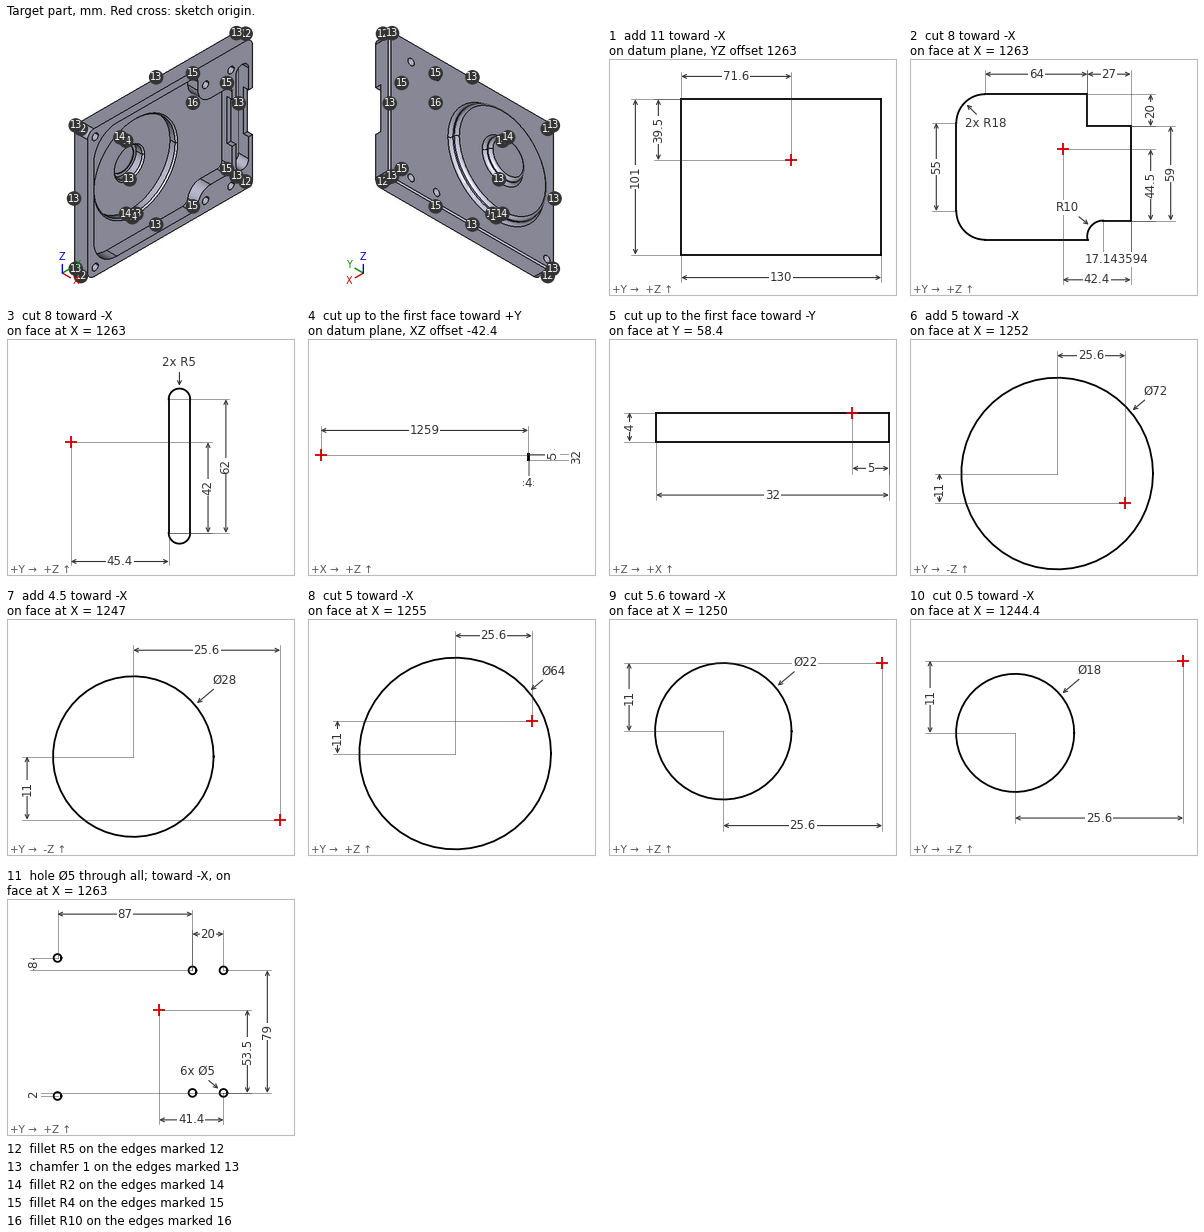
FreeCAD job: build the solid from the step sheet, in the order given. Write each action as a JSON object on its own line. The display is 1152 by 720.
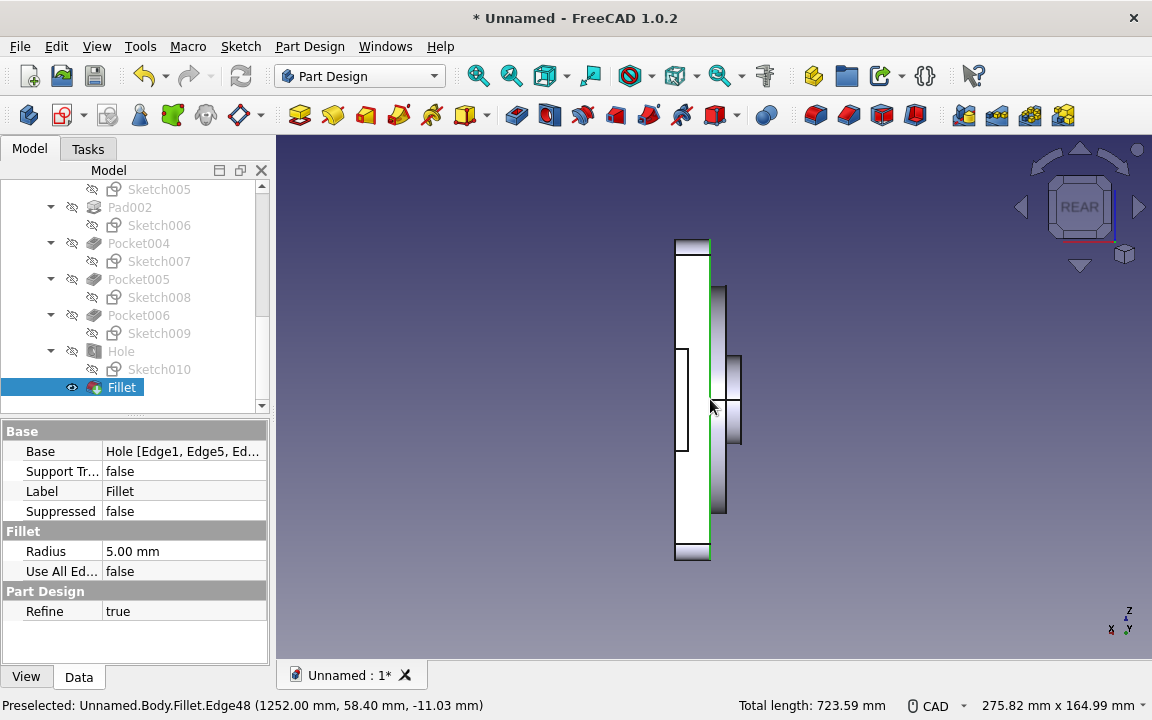
{"action": "left_click", "coordinate": [849, 116]}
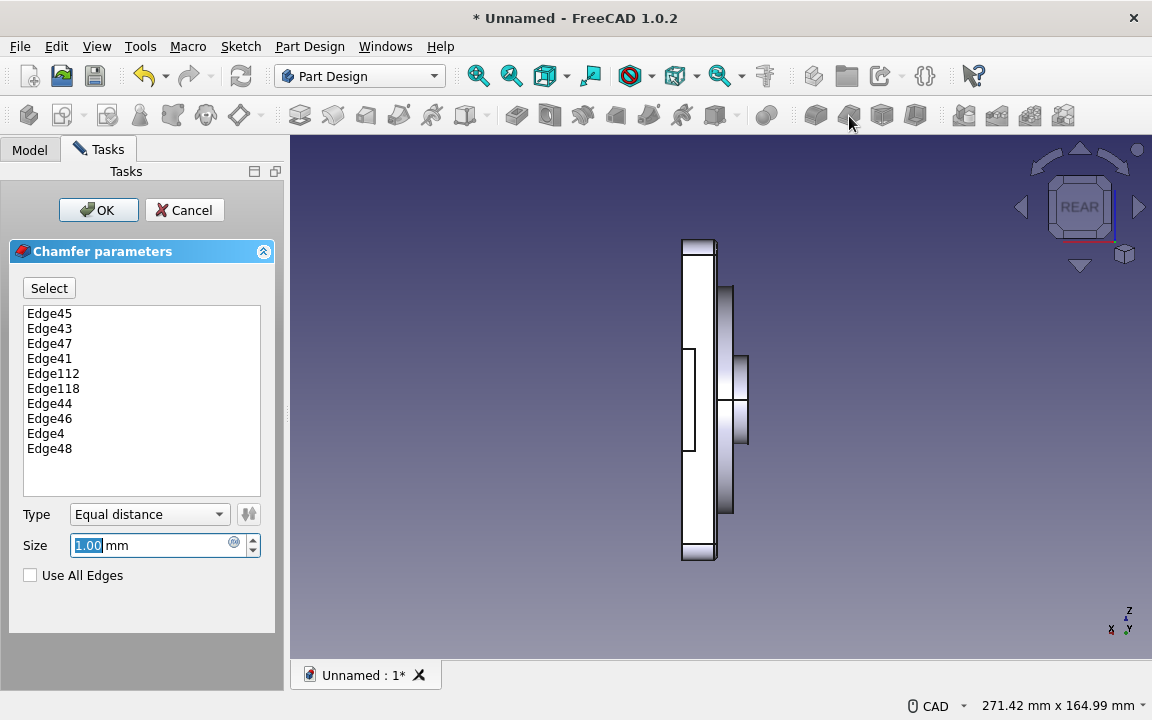
{"action": "type", "text": "1"}
{"action": "key", "text": "Tab"}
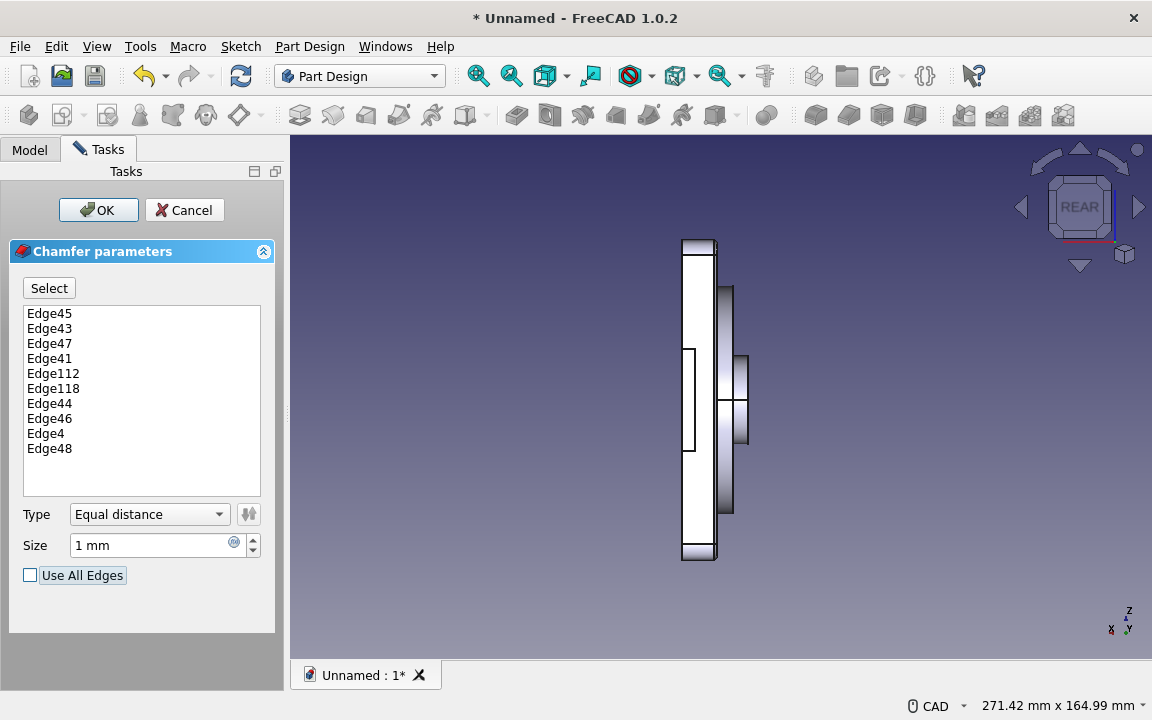
{"action": "left_click", "coordinate": [99, 210]}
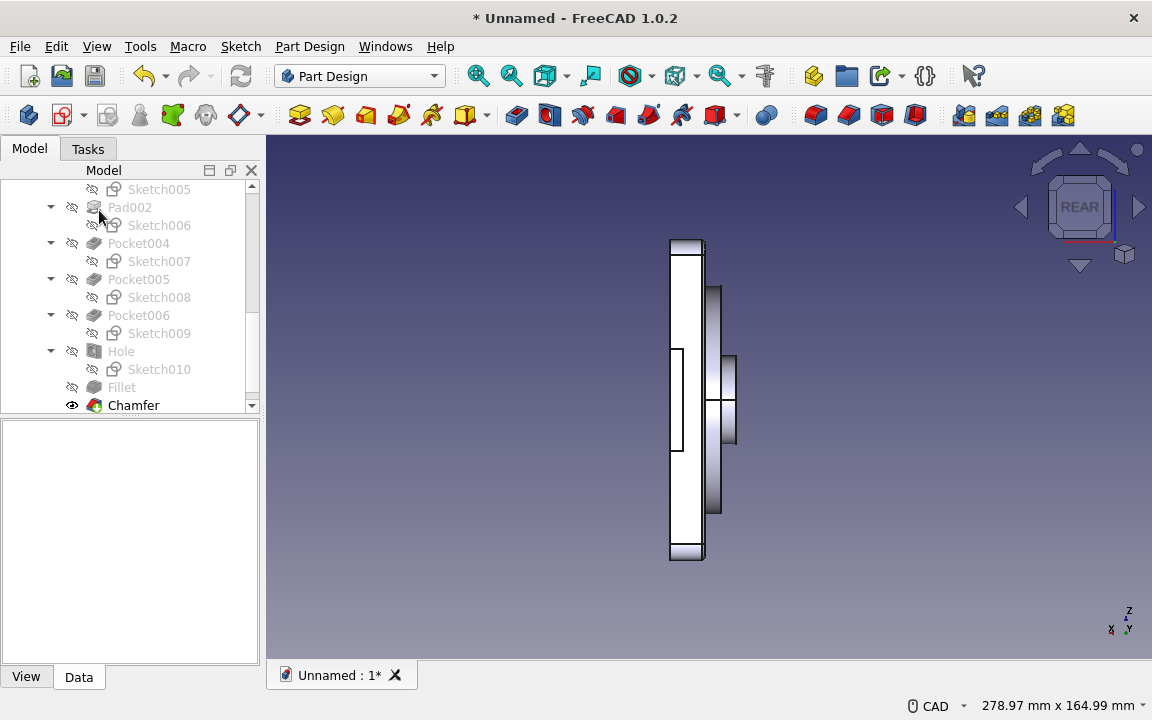
{"action": "left_click", "coordinate": [721, 466]}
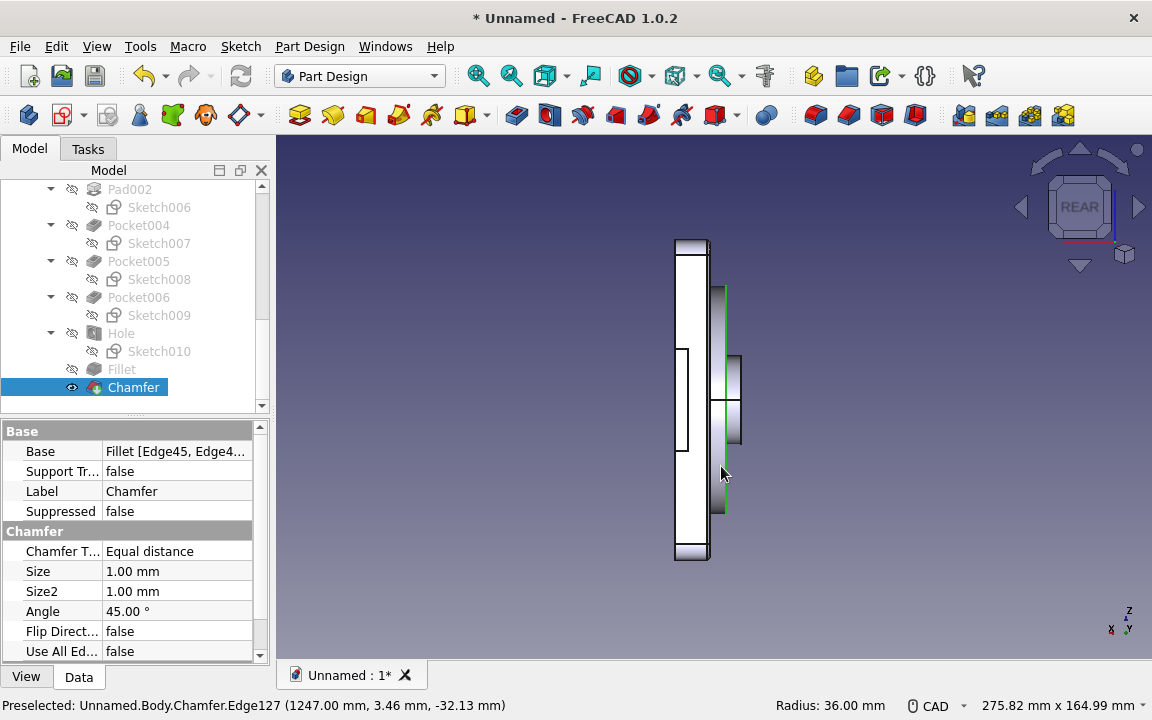
{"action": "left_click", "coordinate": [741, 425], "text": "ctrl"}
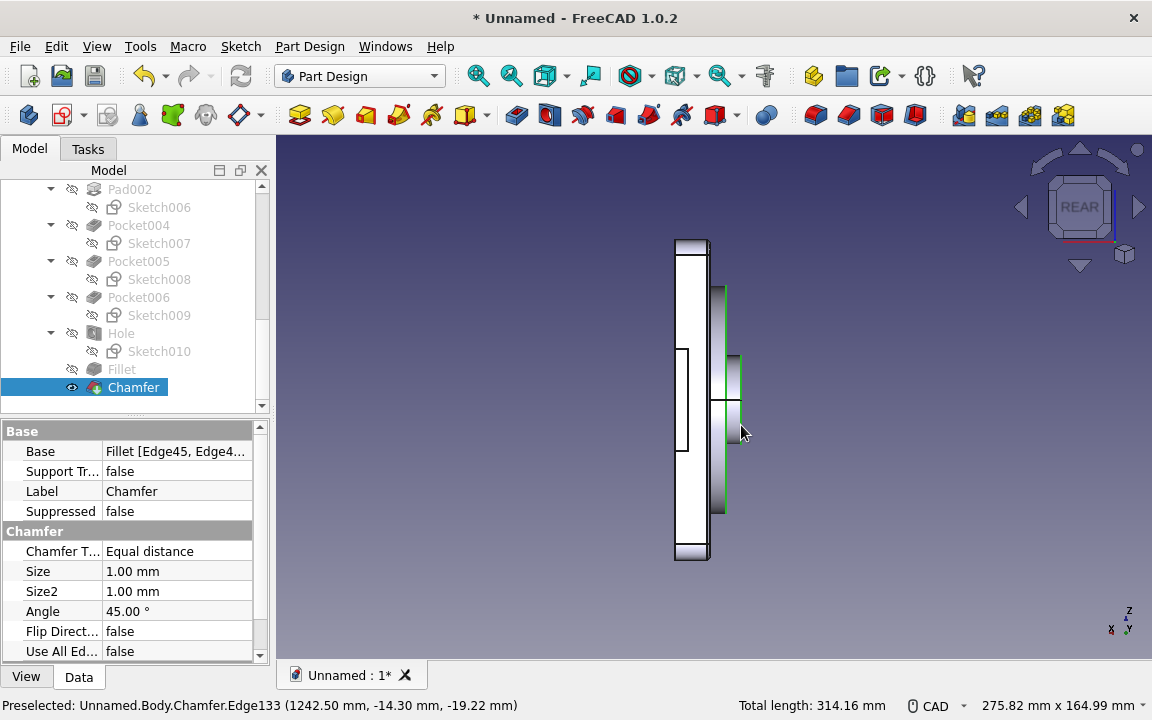
{"action": "key", "text": "0"}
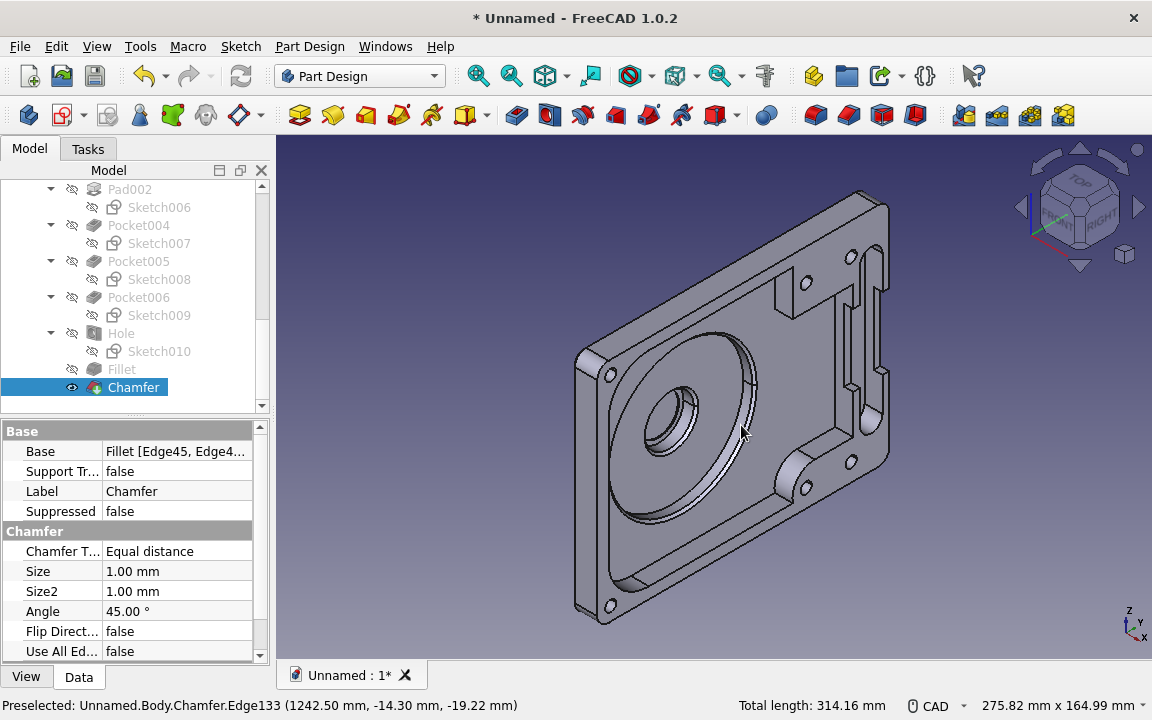
{"action": "key", "text": "2"}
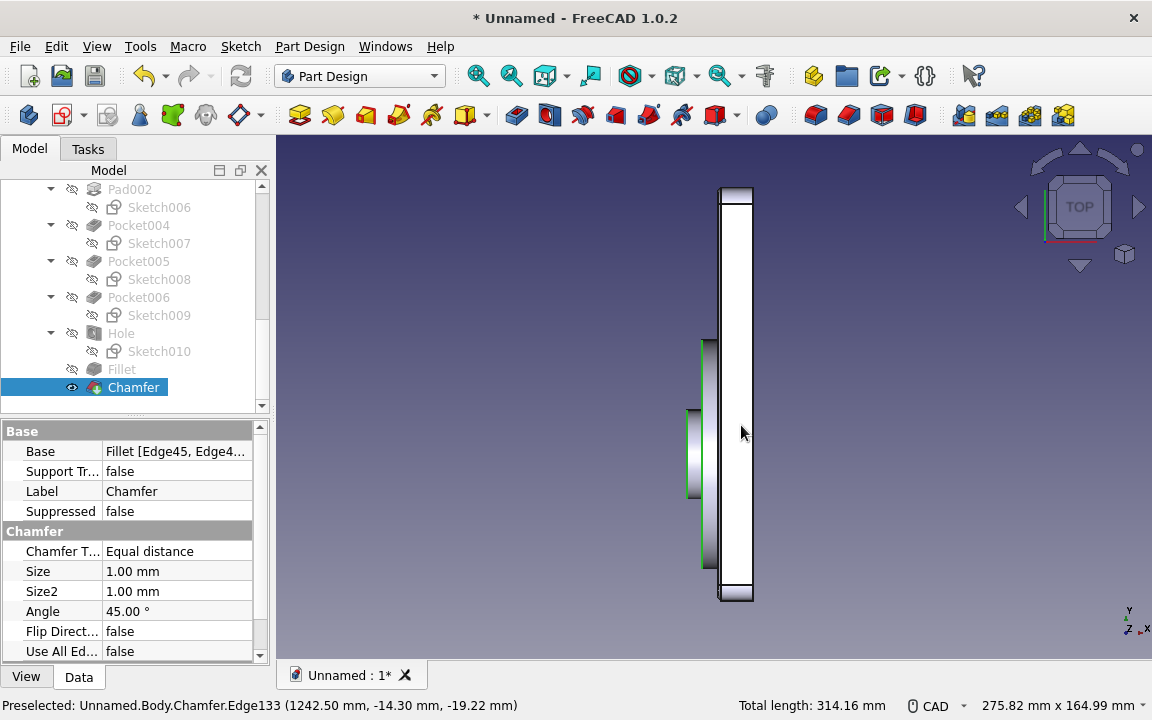
{"action": "key", "text": "1"}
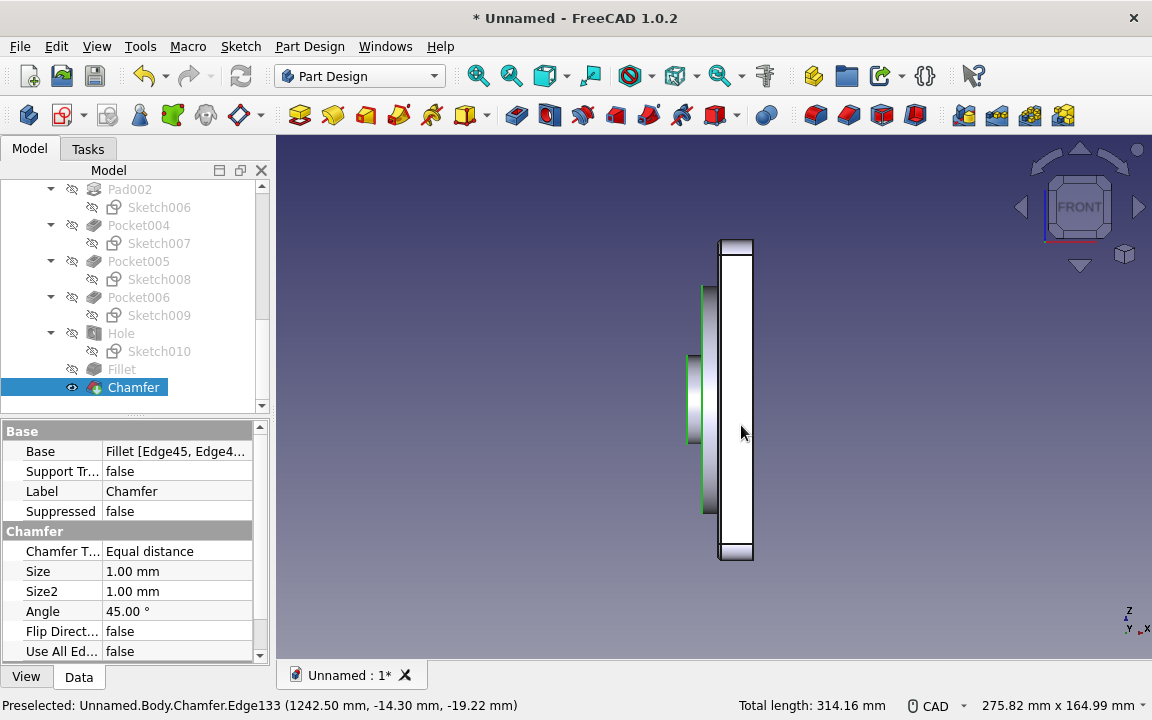
{"action": "key", "text": "3"}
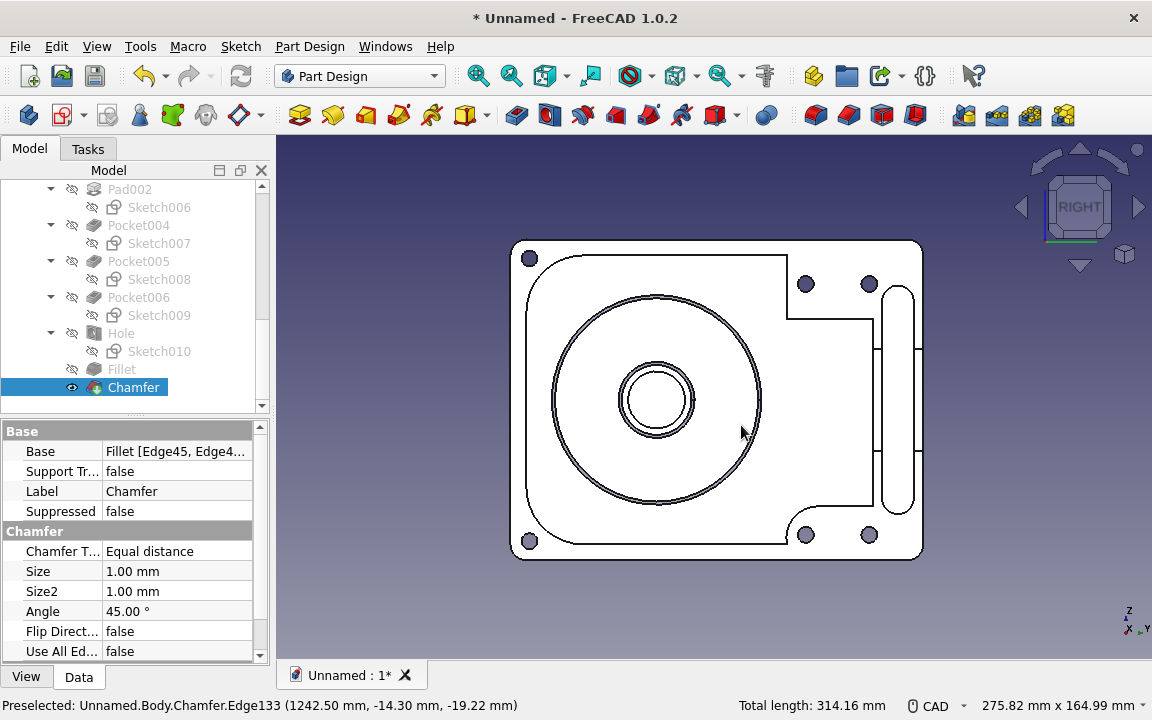
{"action": "key", "text": "5"}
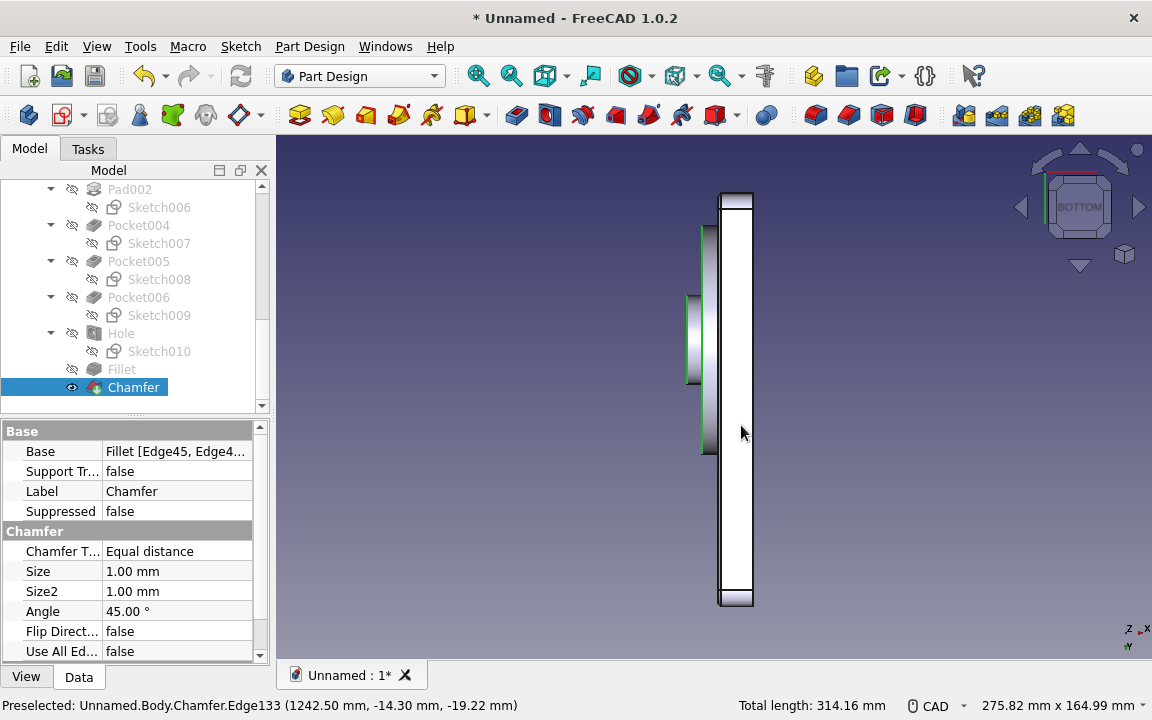
{"action": "key", "text": "4"}